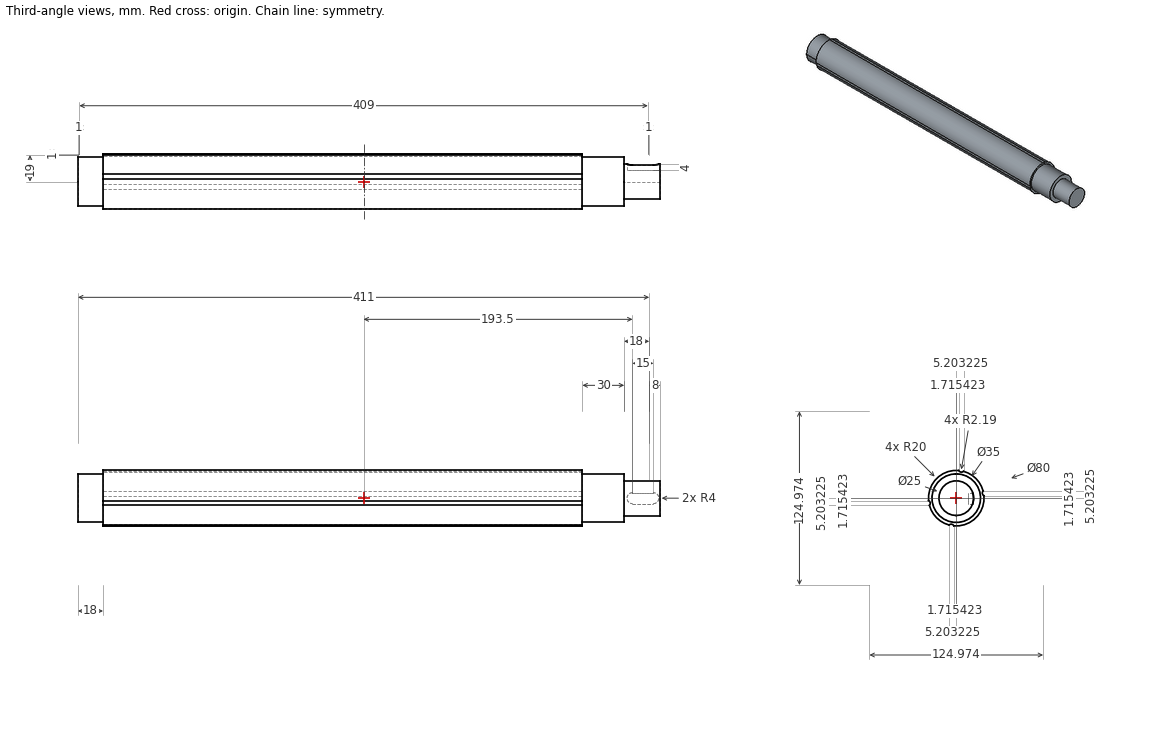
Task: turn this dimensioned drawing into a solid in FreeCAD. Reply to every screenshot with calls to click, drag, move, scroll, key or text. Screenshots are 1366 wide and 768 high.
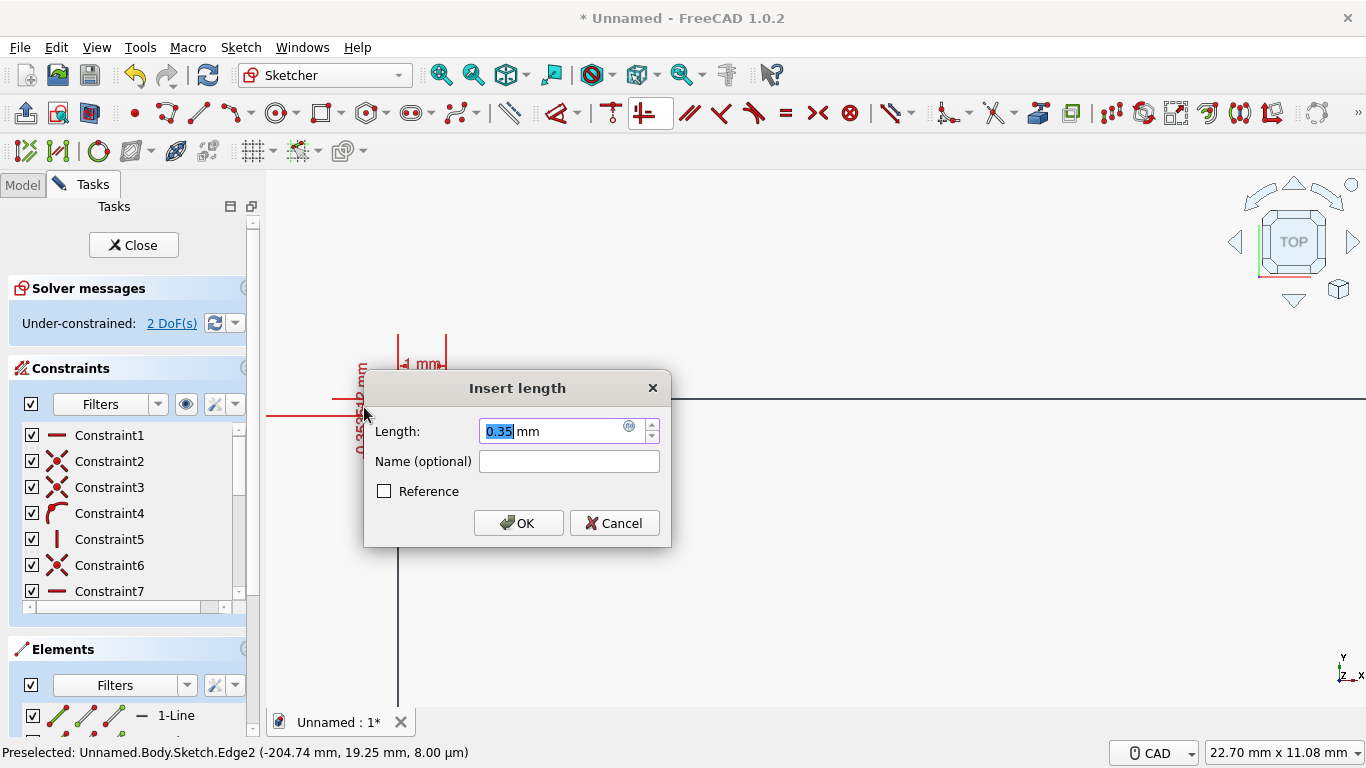
text(1)
key(Return)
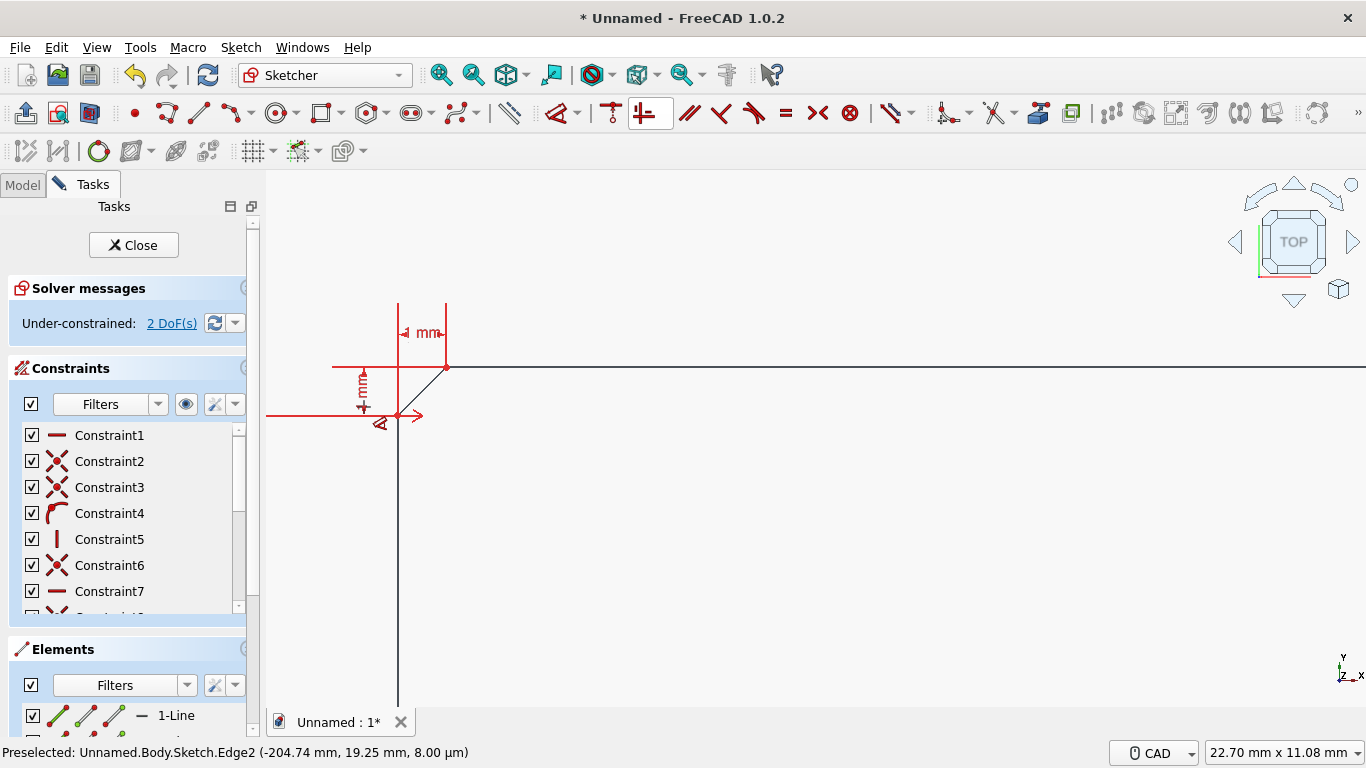
scroll(339, 421, down, 16)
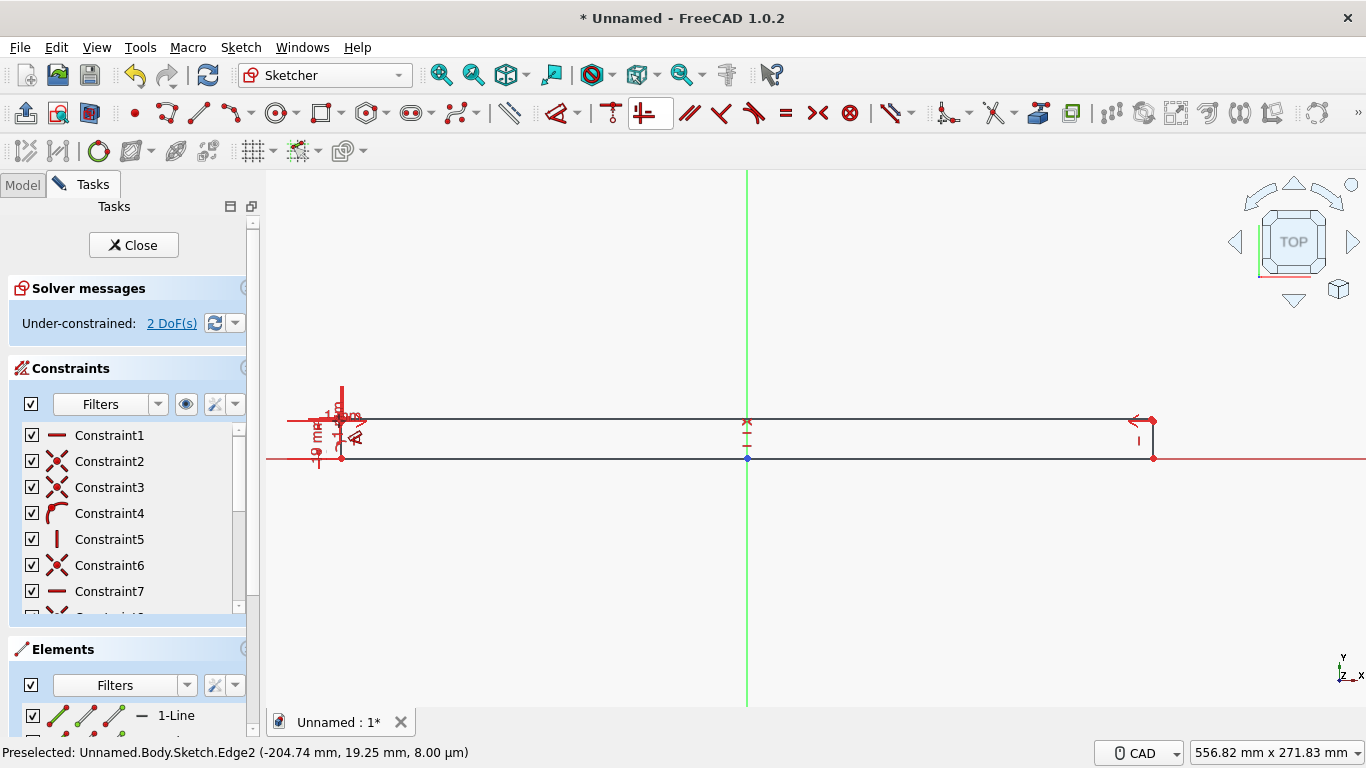
scroll(1153, 421, up, 16)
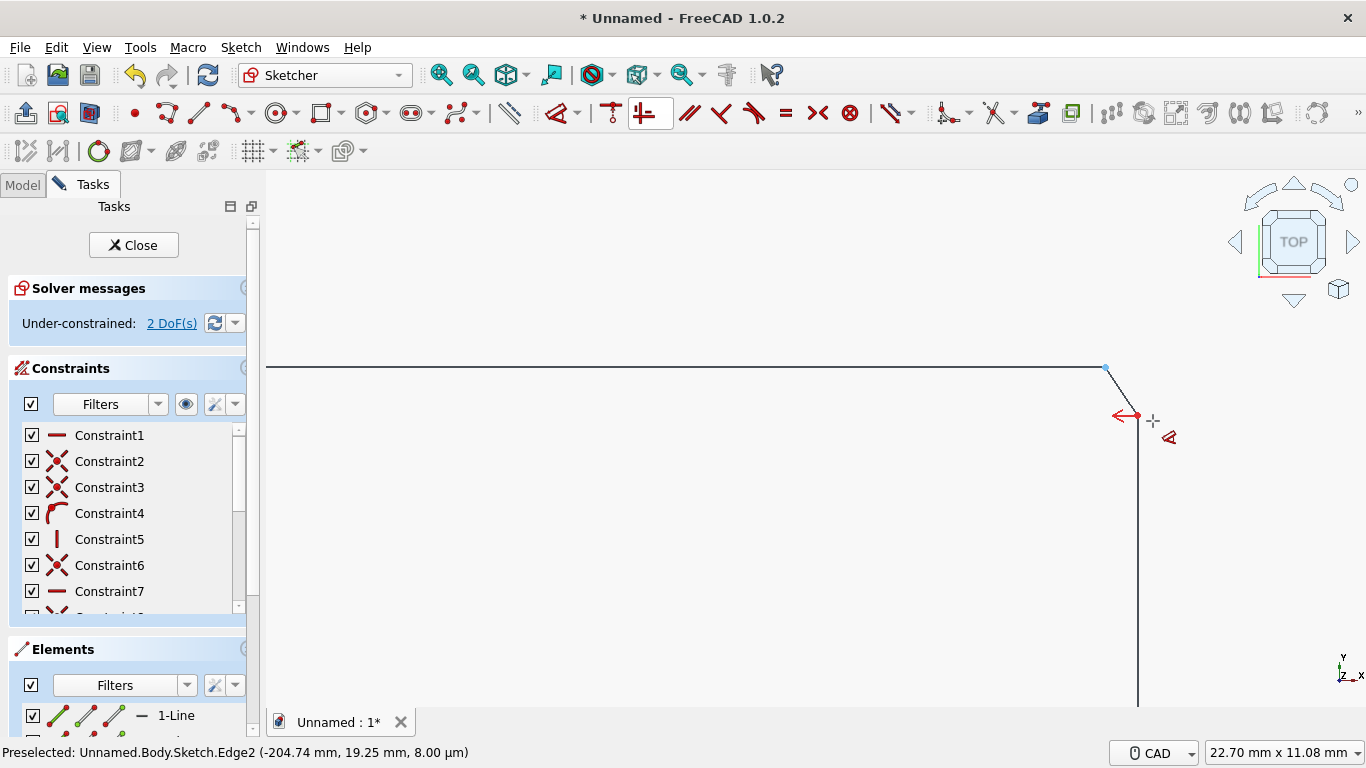
click(1128, 401)
click(1121, 333)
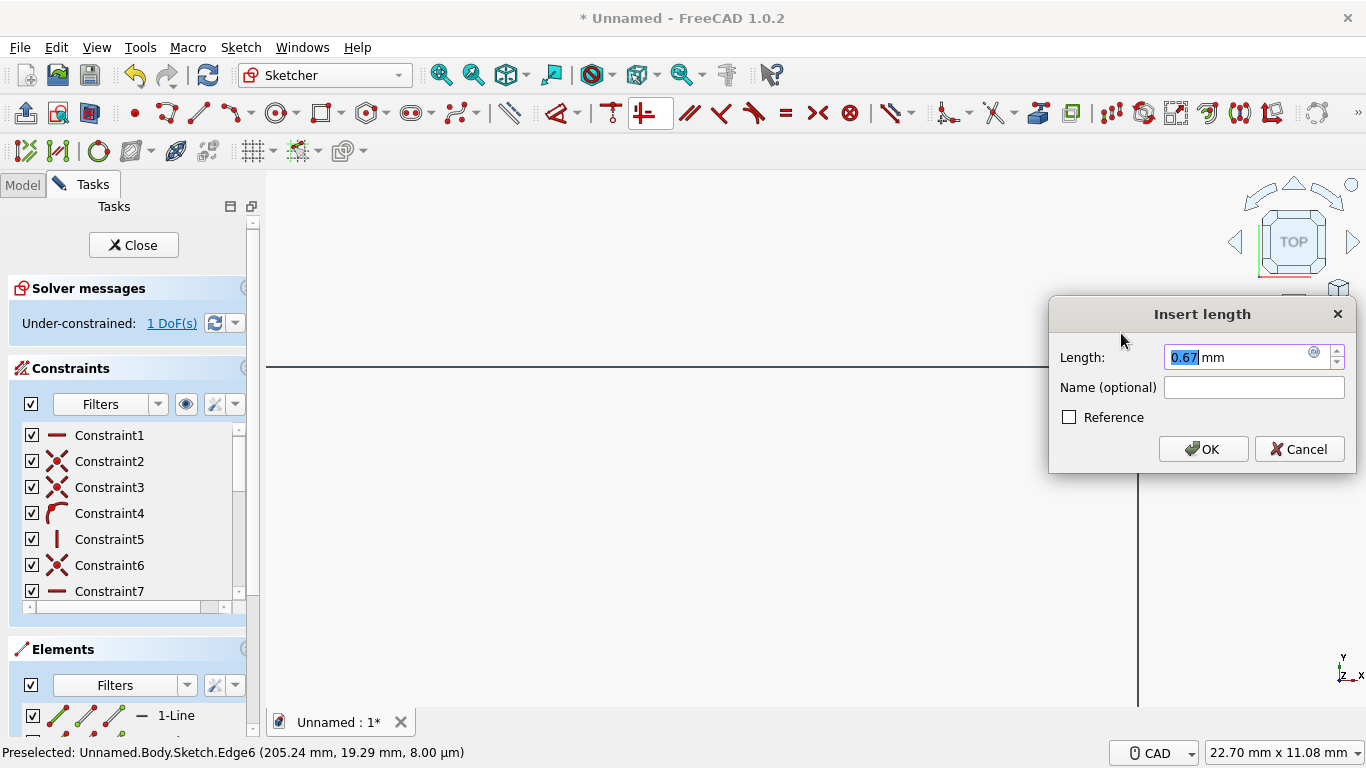
text(1)
key(Return)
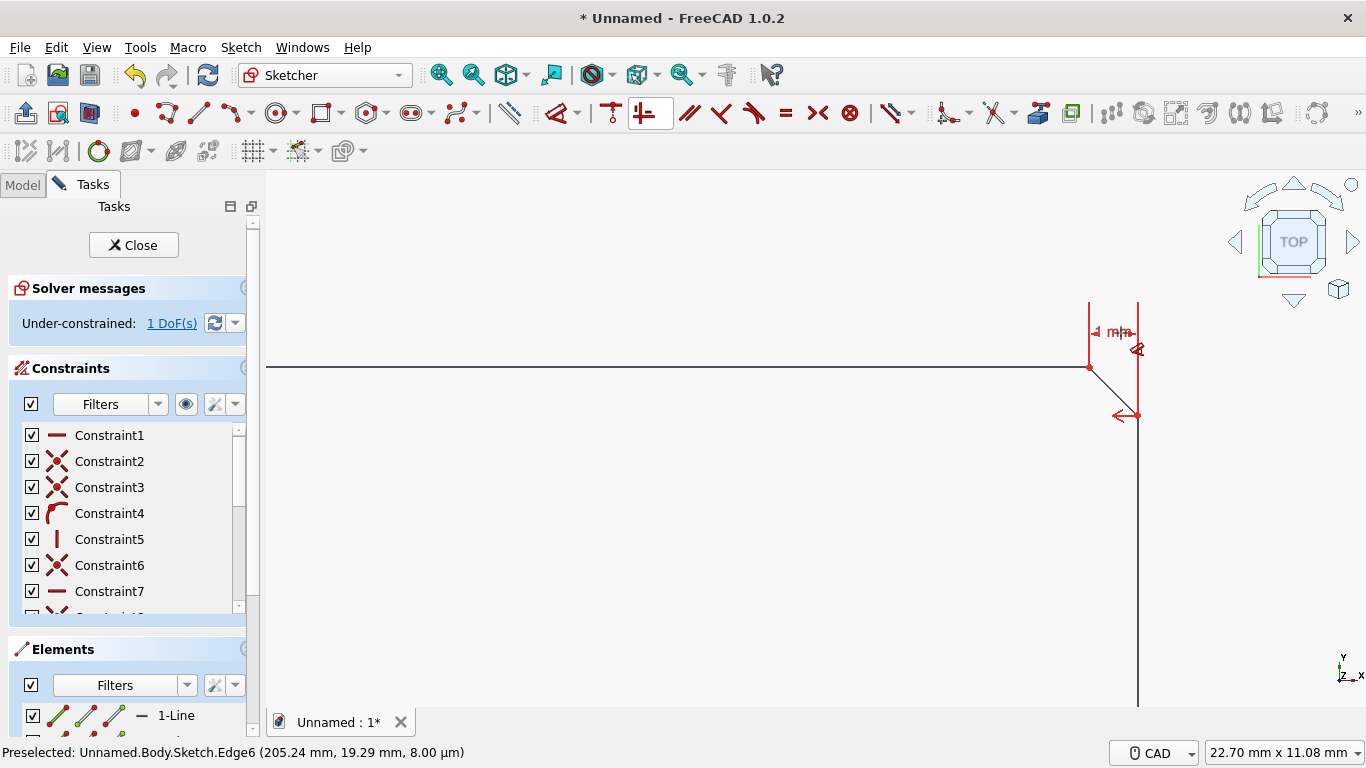
scroll(1154, 421, down, 16)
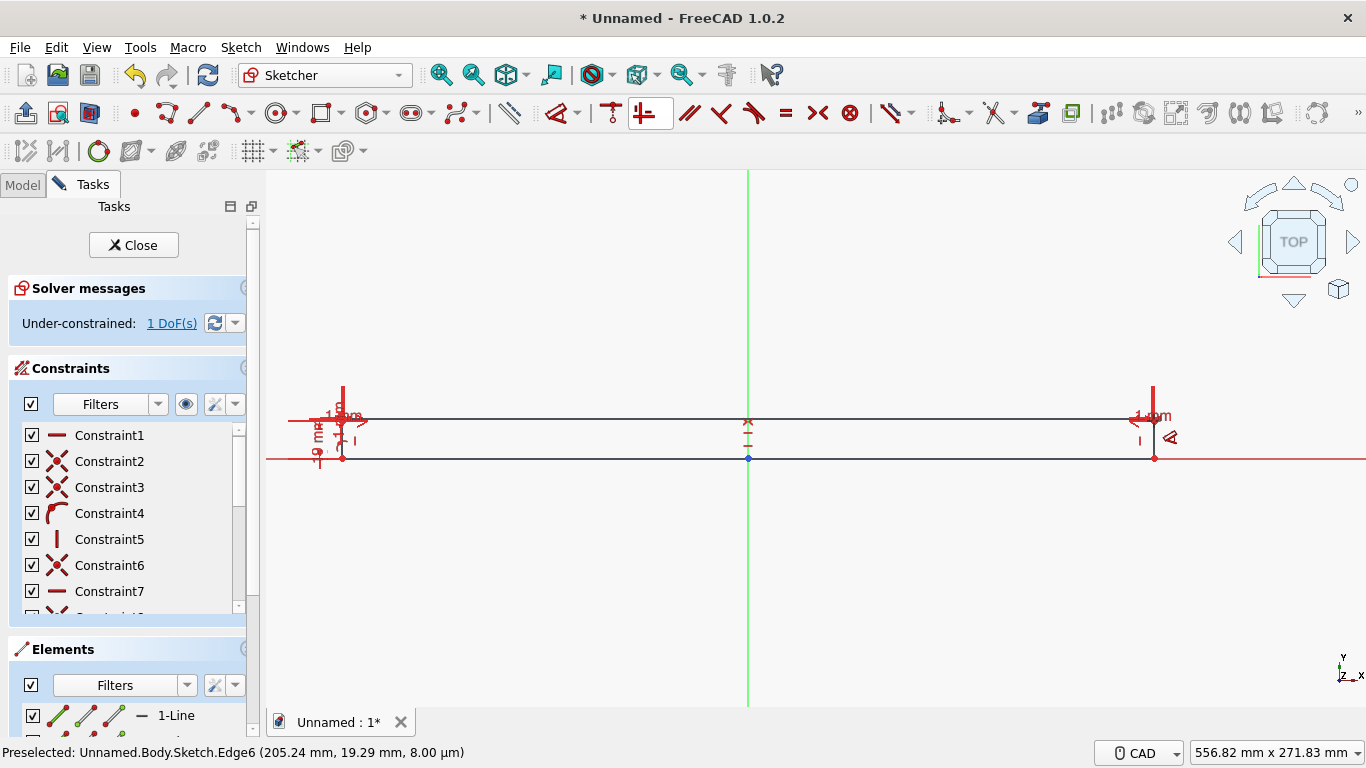
click(910, 419)
click(562, 385)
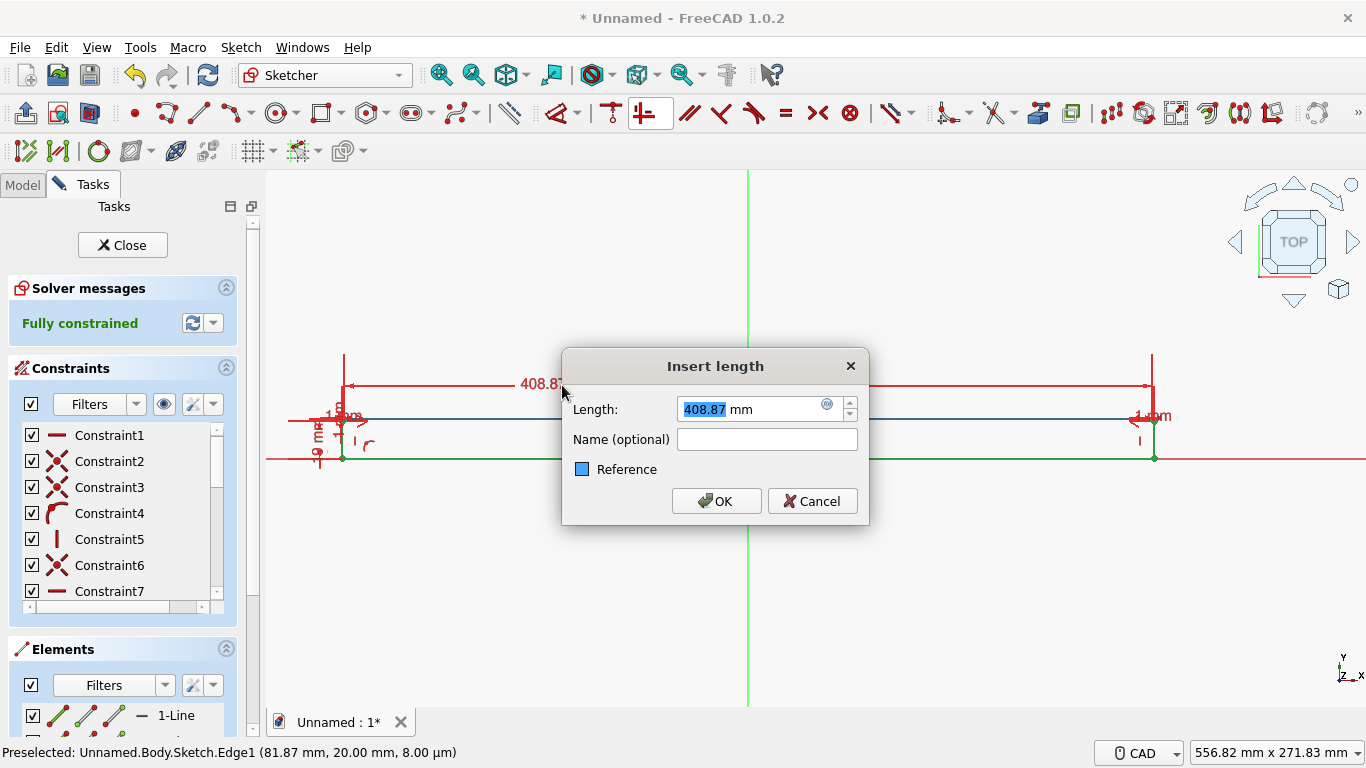
text(409)
key(Return)
key(Escape)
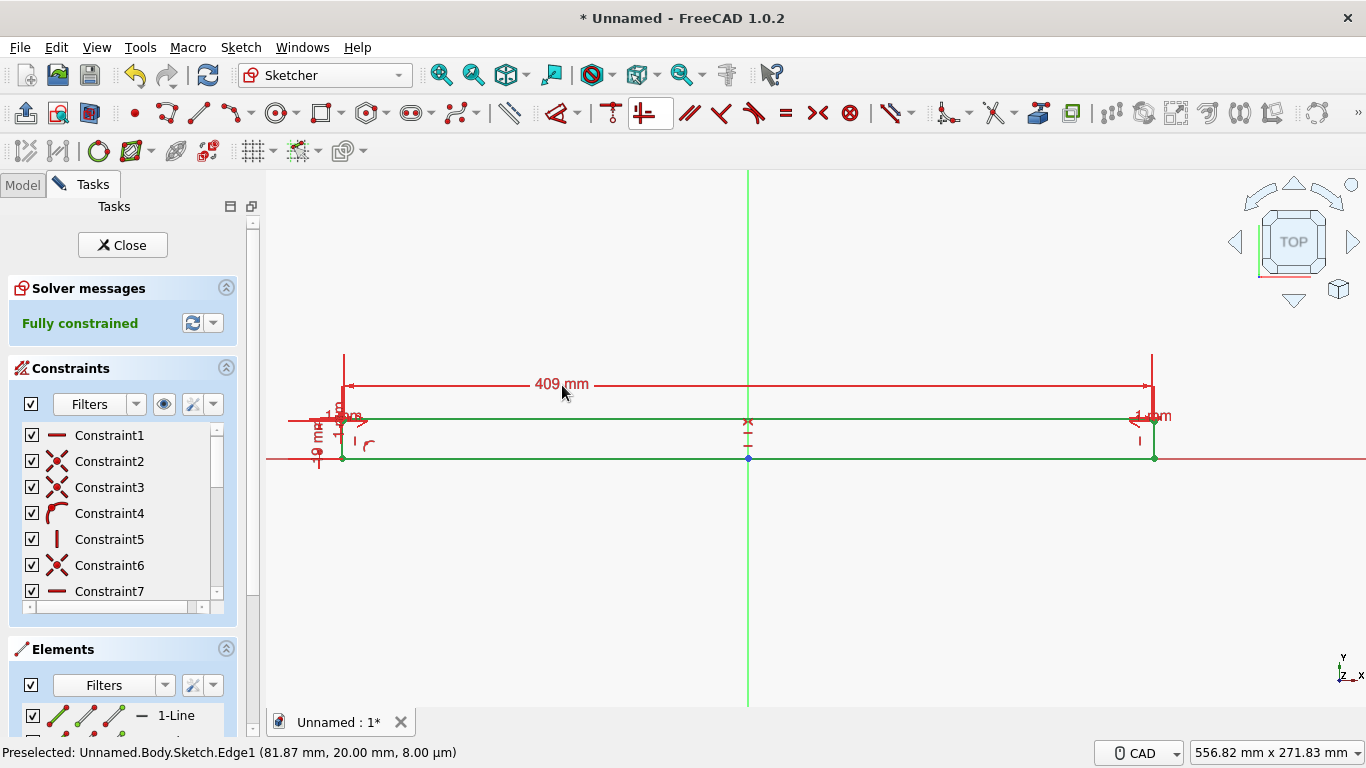
click(123, 245)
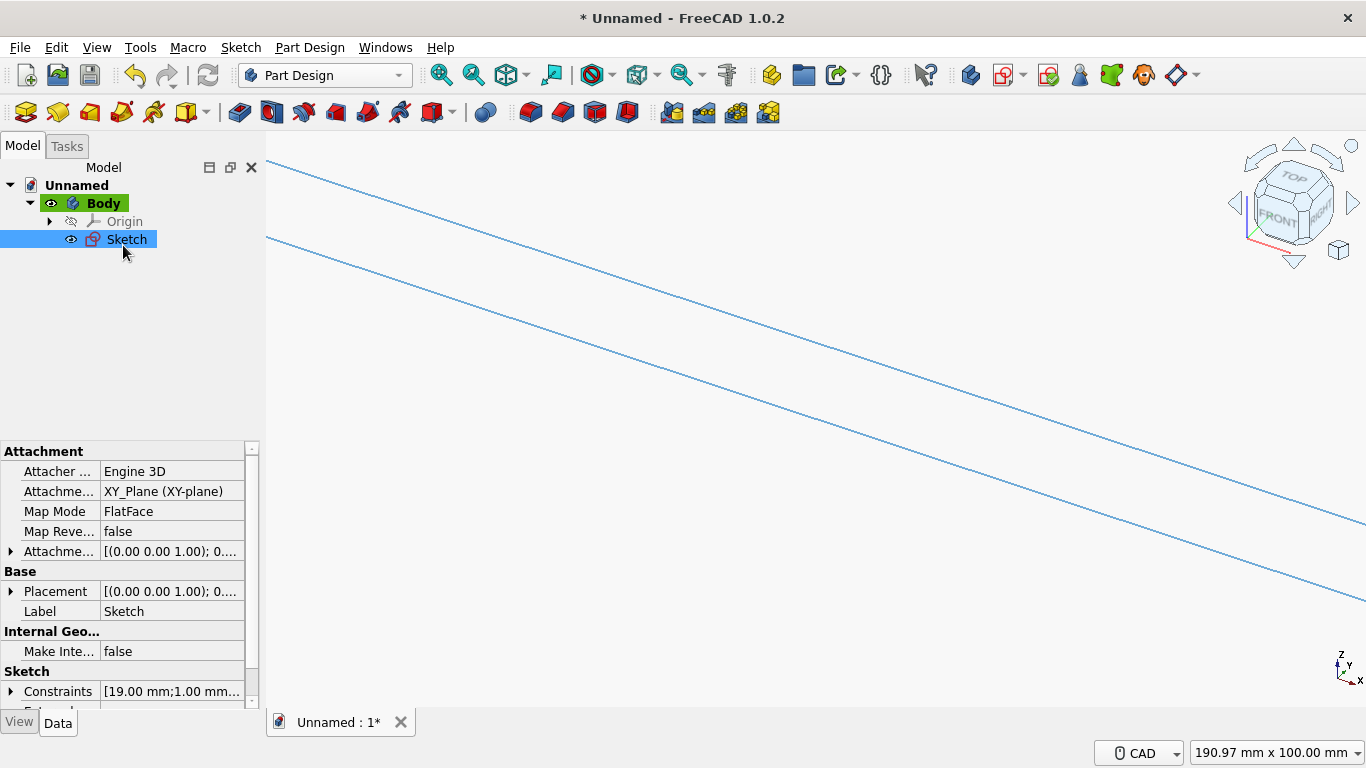
click(58, 112)